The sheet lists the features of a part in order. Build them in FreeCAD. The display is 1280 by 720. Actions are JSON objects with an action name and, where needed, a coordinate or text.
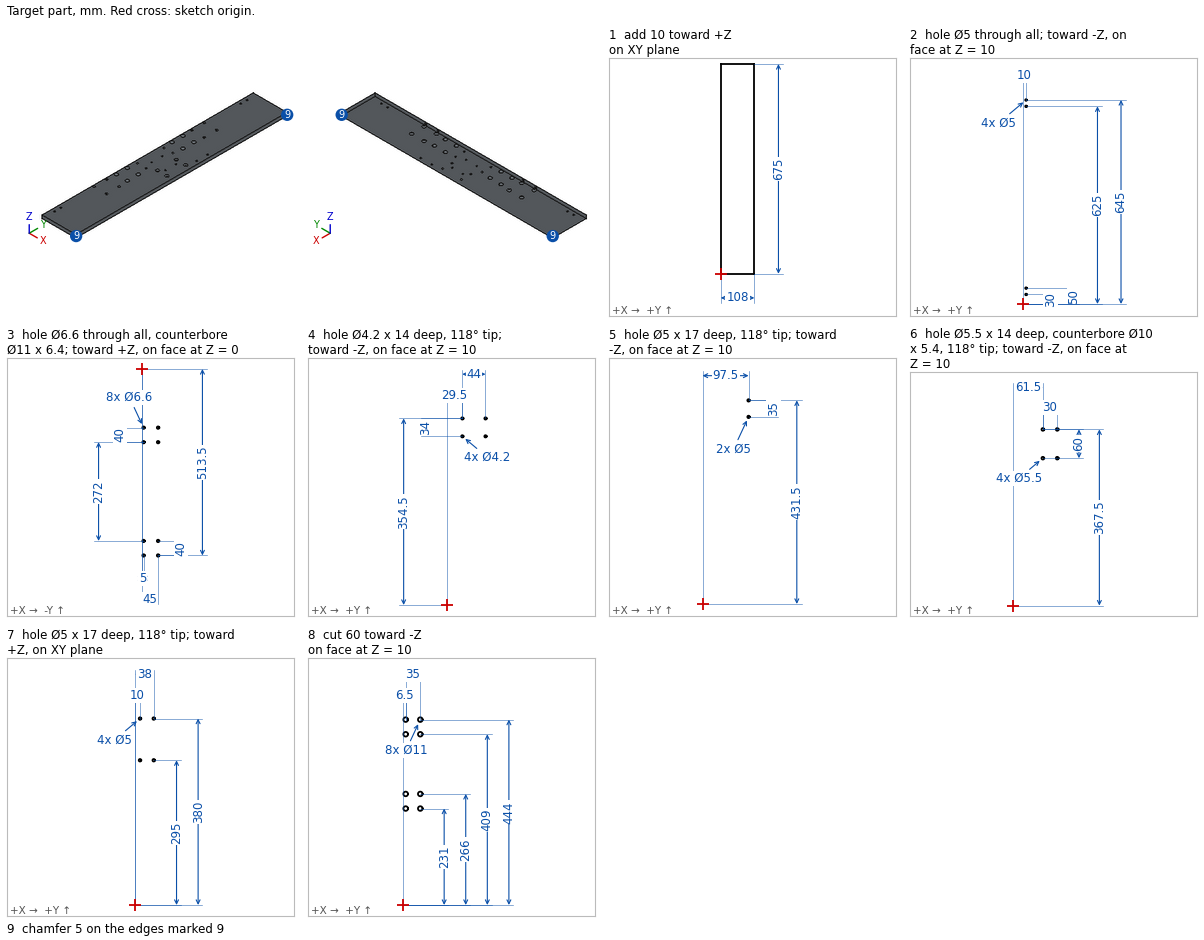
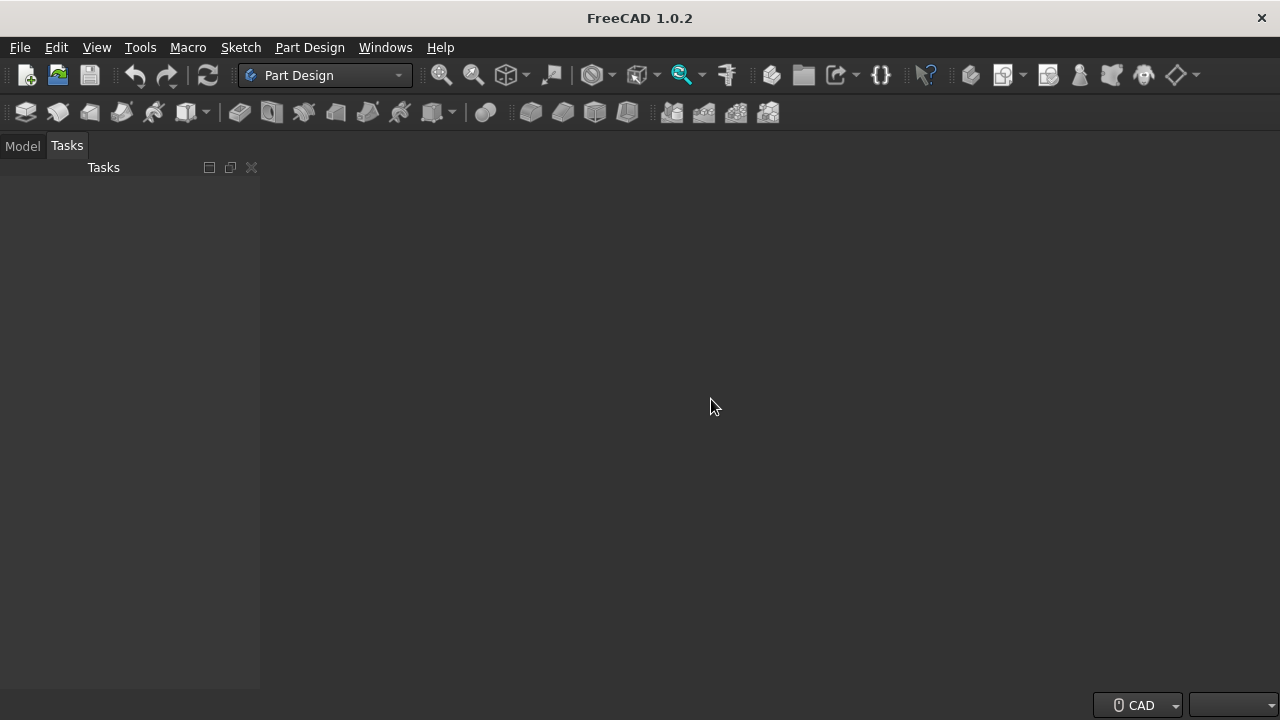
{"action": "left_click", "coordinate": [26, 76]}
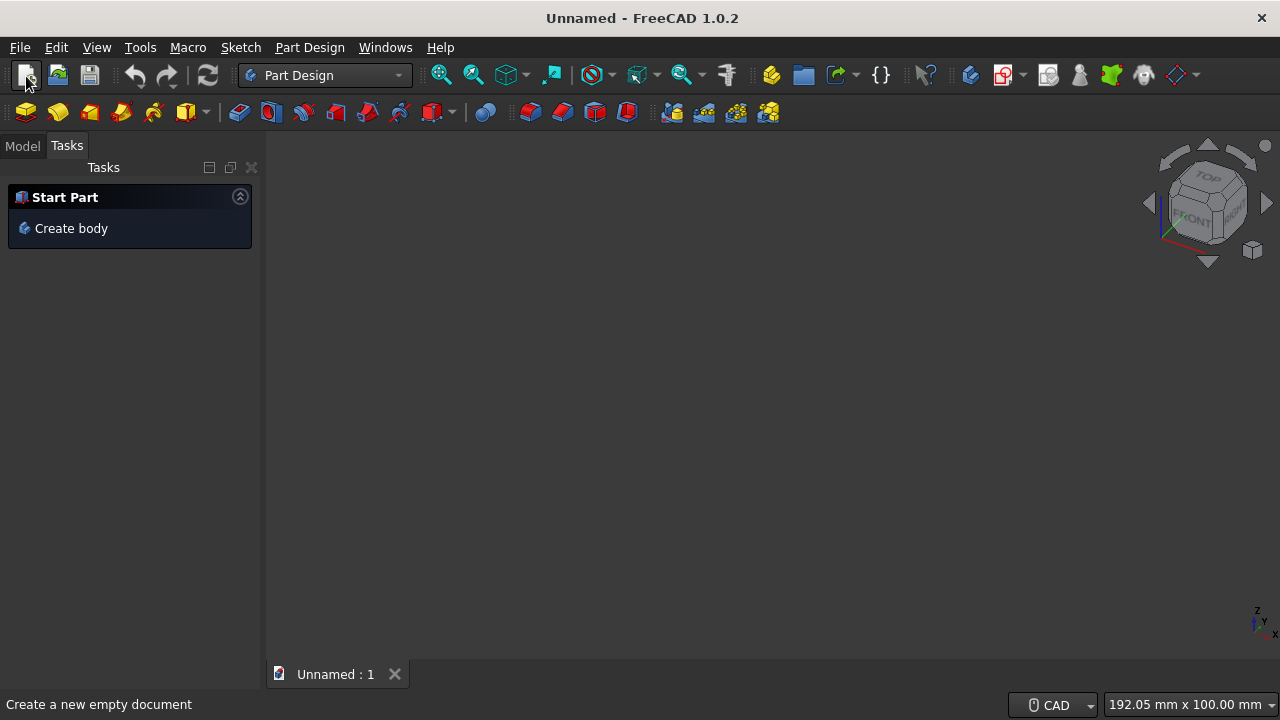
{"action": "left_click", "coordinate": [1004, 76]}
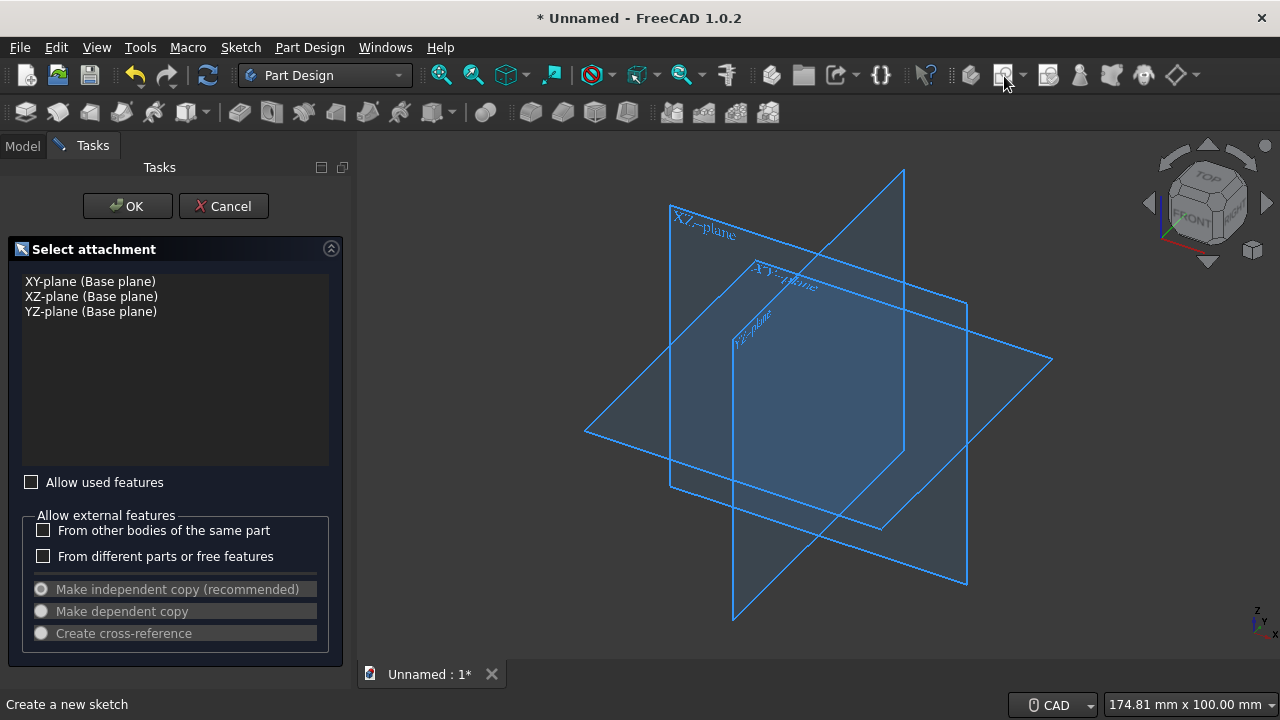
{"action": "left_click", "coordinate": [82, 282]}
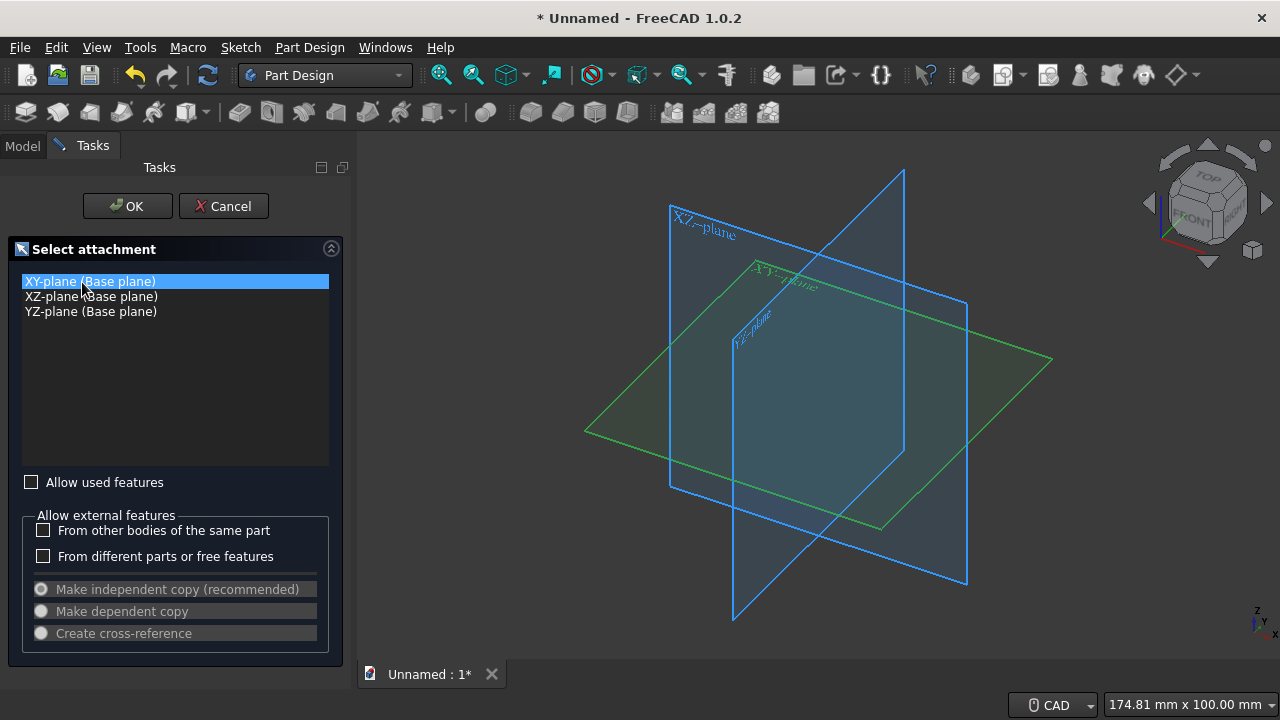
{"action": "left_click", "coordinate": [128, 206]}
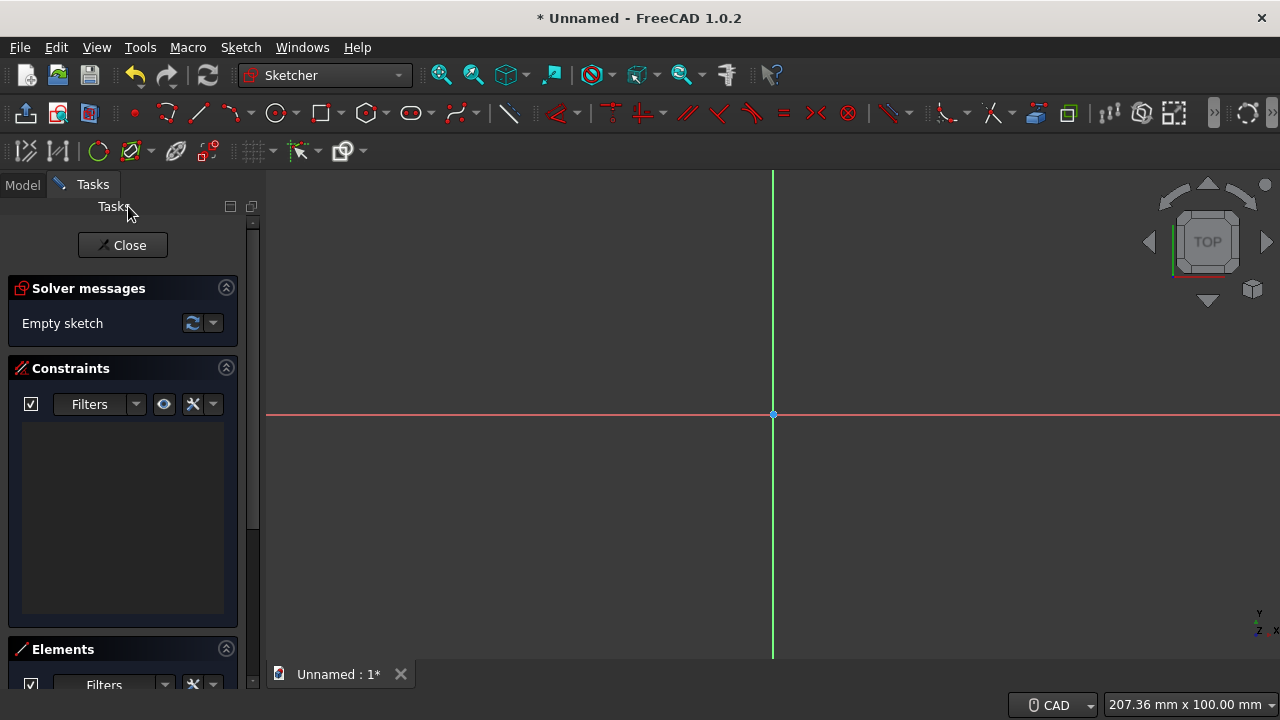
{"action": "scroll", "coordinate": [671, 579], "scroll_direction": "down", "scroll_amount": 12}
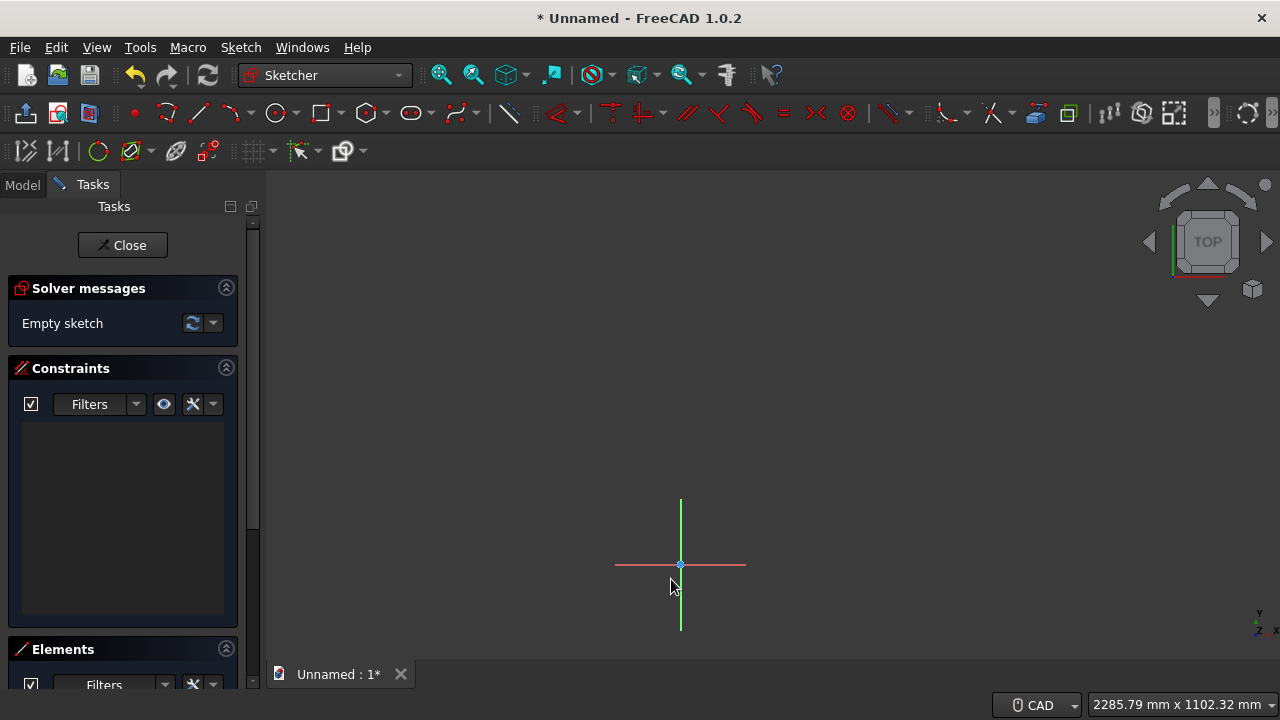
{"action": "left_click", "coordinate": [322, 114]}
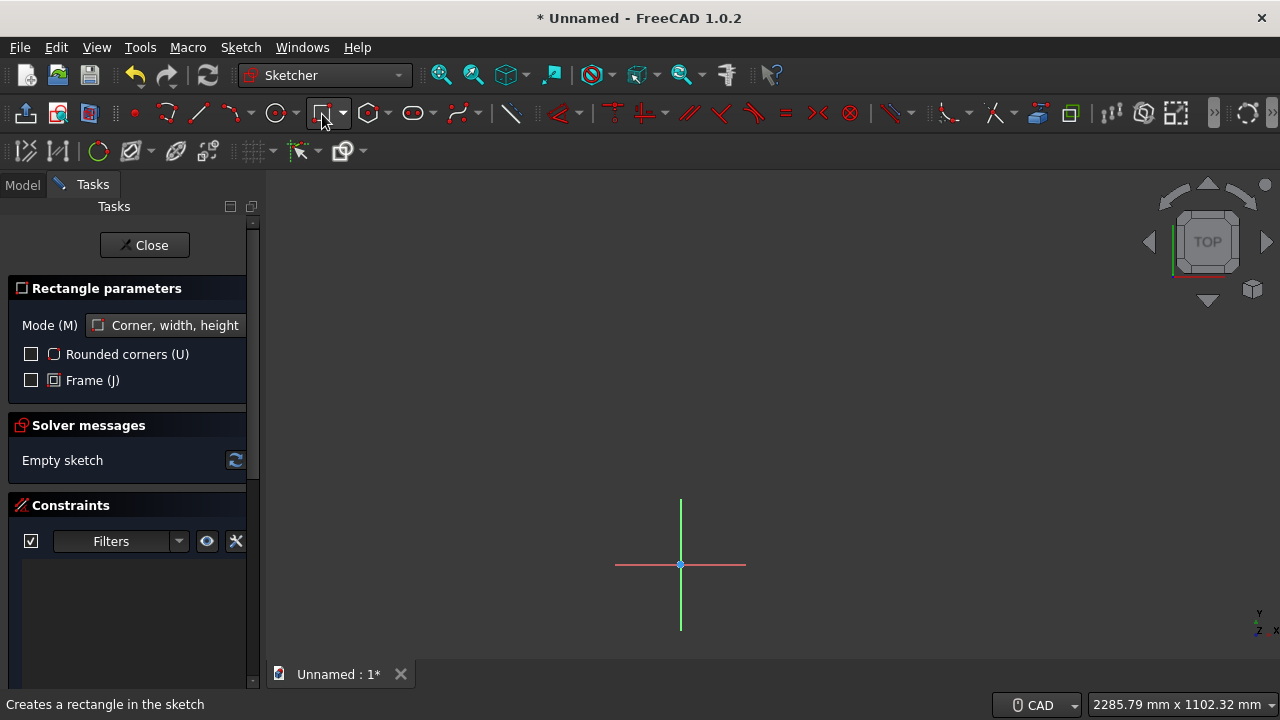
{"action": "left_click", "coordinate": [681, 565]}
{"action": "mouse_move", "coordinate": [729, 265]}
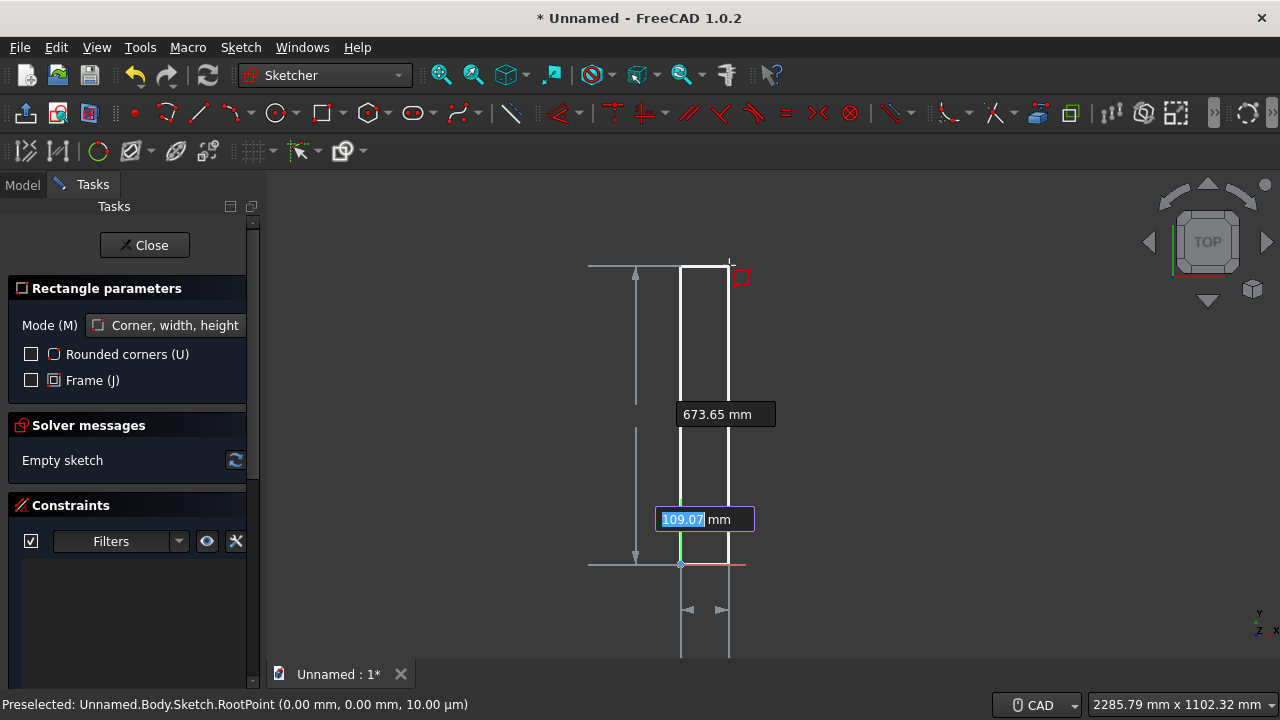
{"action": "type", "text": "108"}
{"action": "key", "text": "Tab"}
{"action": "type", "text": "675"}
{"action": "key", "text": "Return"}
{"action": "key", "text": "Escape"}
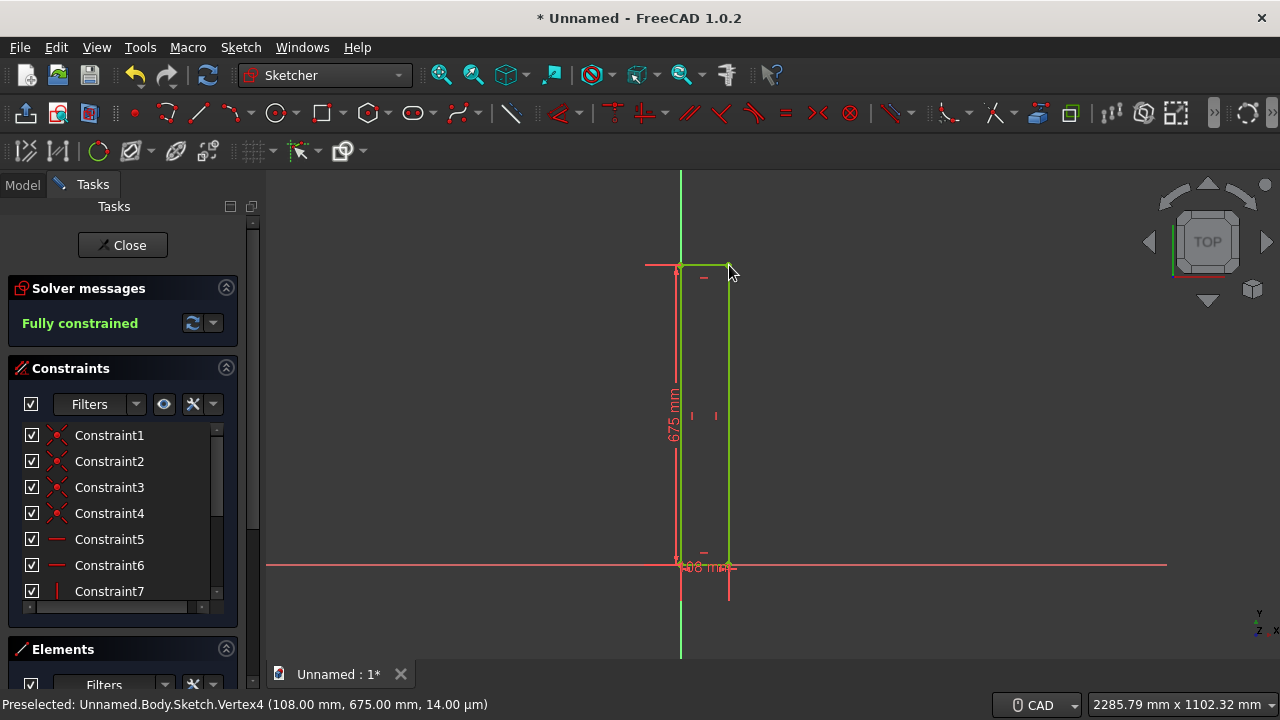
{"action": "left_click", "coordinate": [123, 245]}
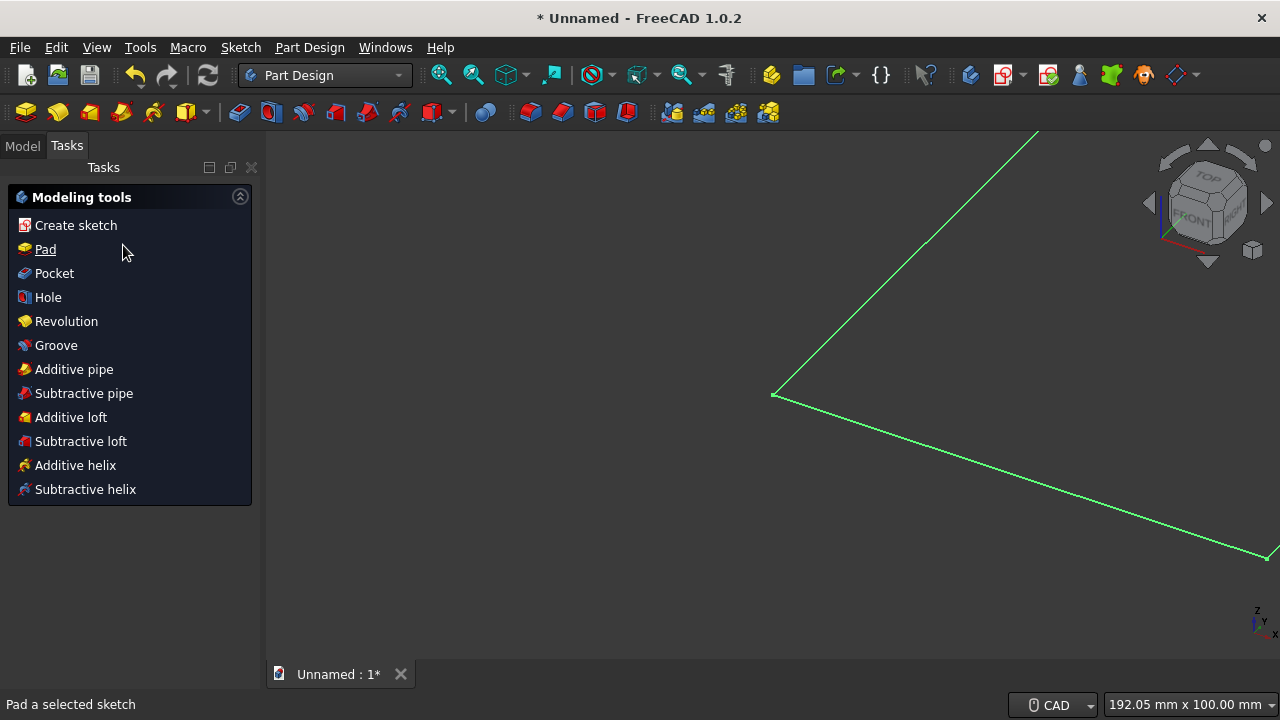
{"action": "left_click", "coordinate": [26, 112]}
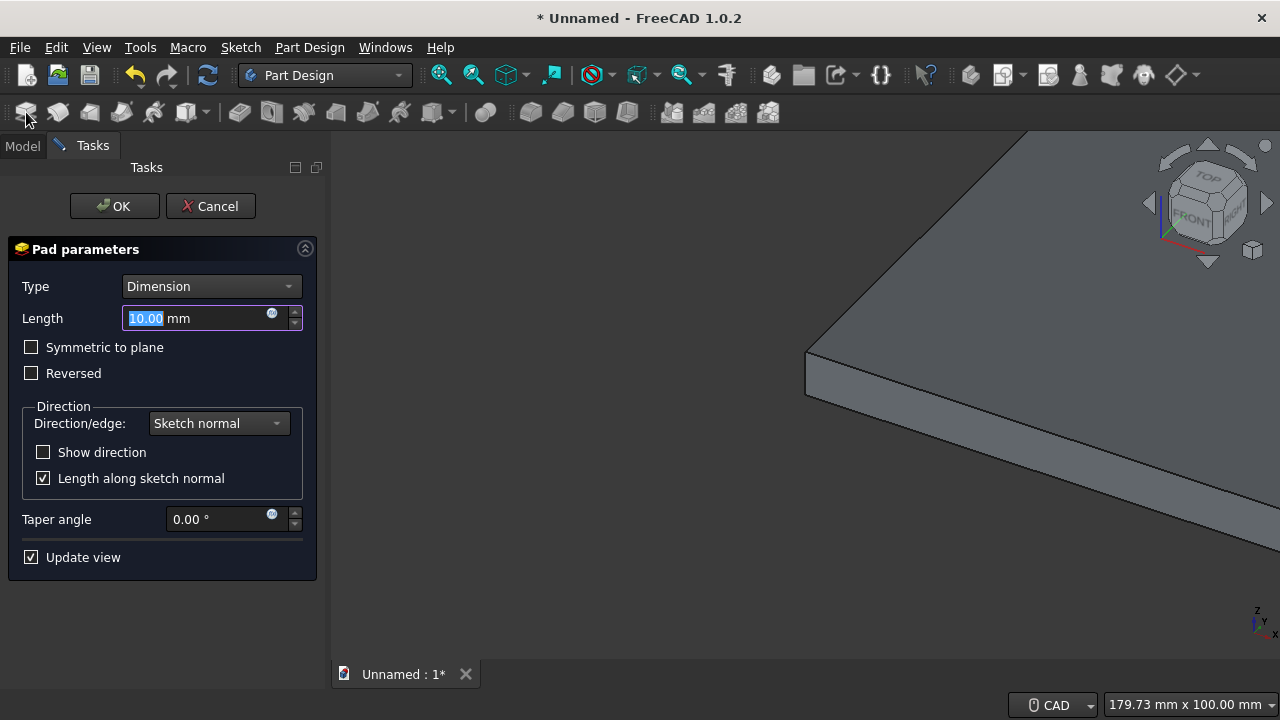
{"action": "type", "text": "10"}
{"action": "key", "text": "Tab"}